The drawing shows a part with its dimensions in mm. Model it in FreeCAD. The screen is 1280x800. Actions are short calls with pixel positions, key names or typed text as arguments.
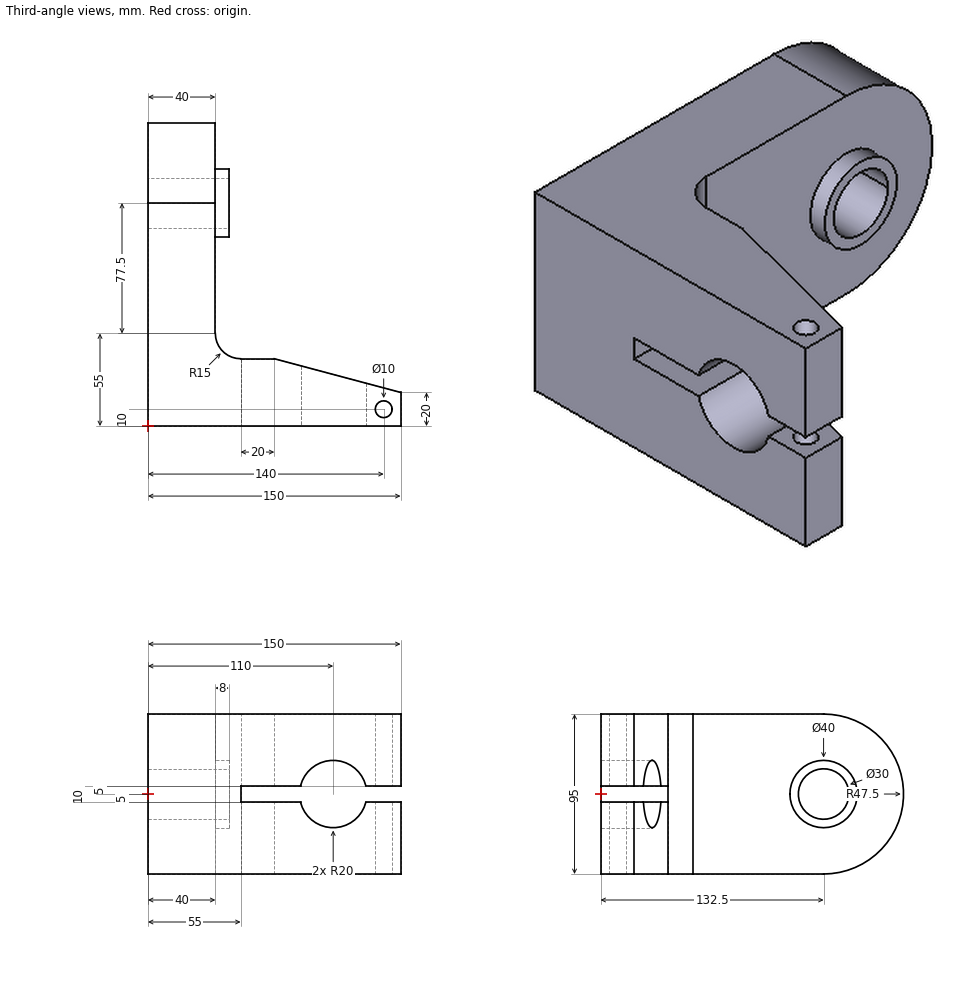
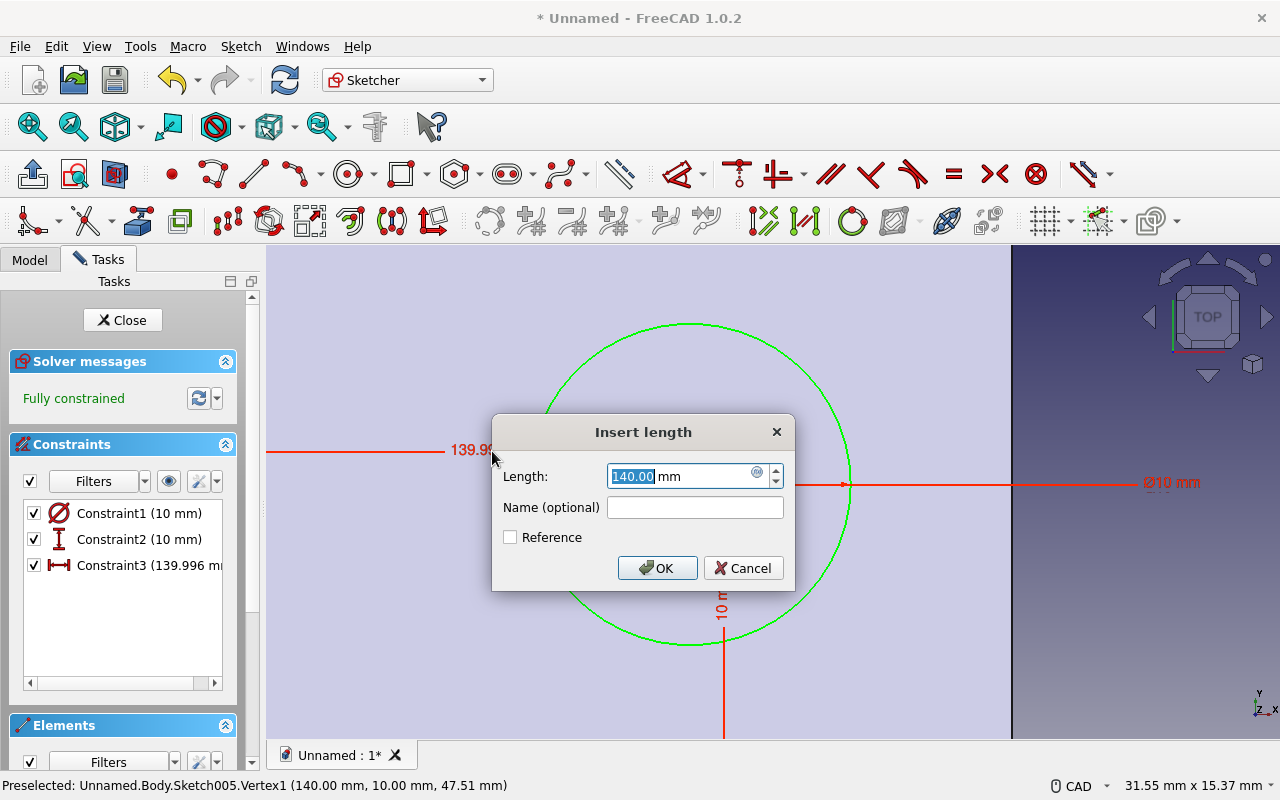
text(140)
key(Return)
key(Escape)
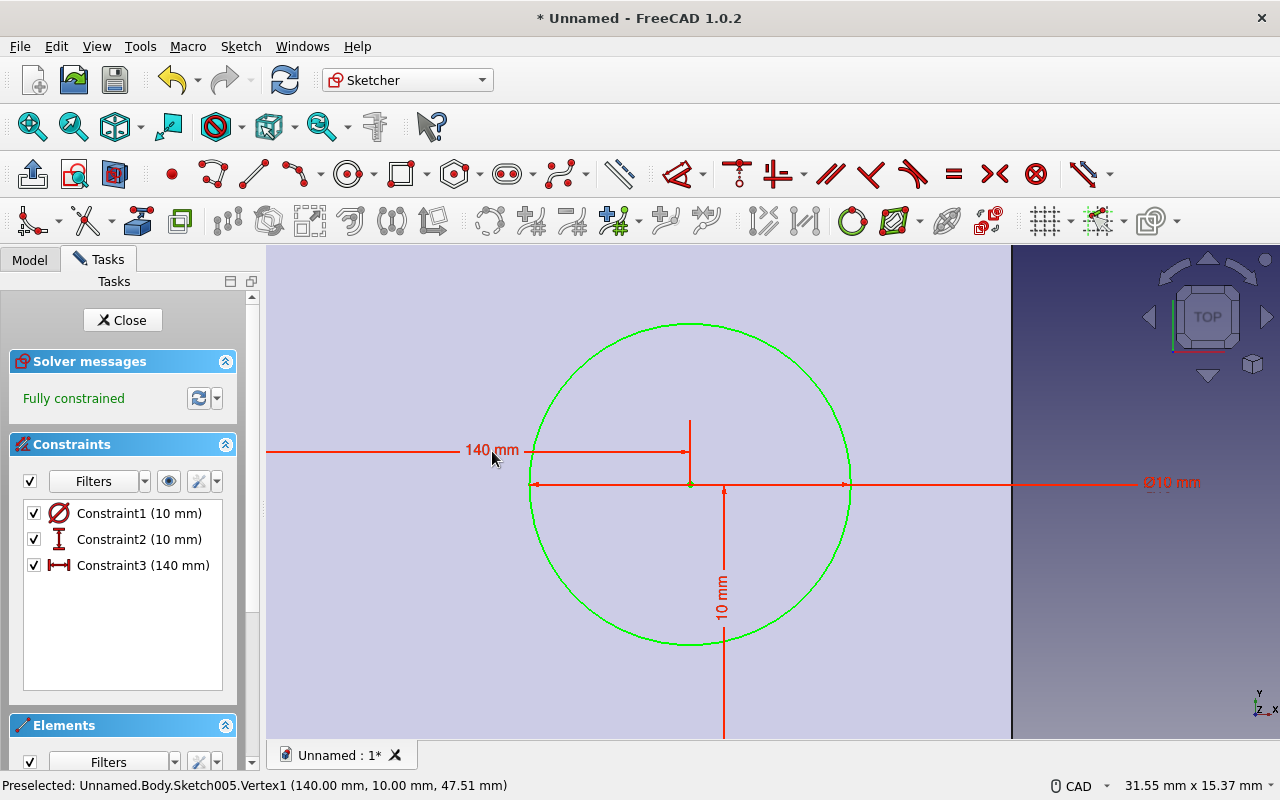
click(123, 320)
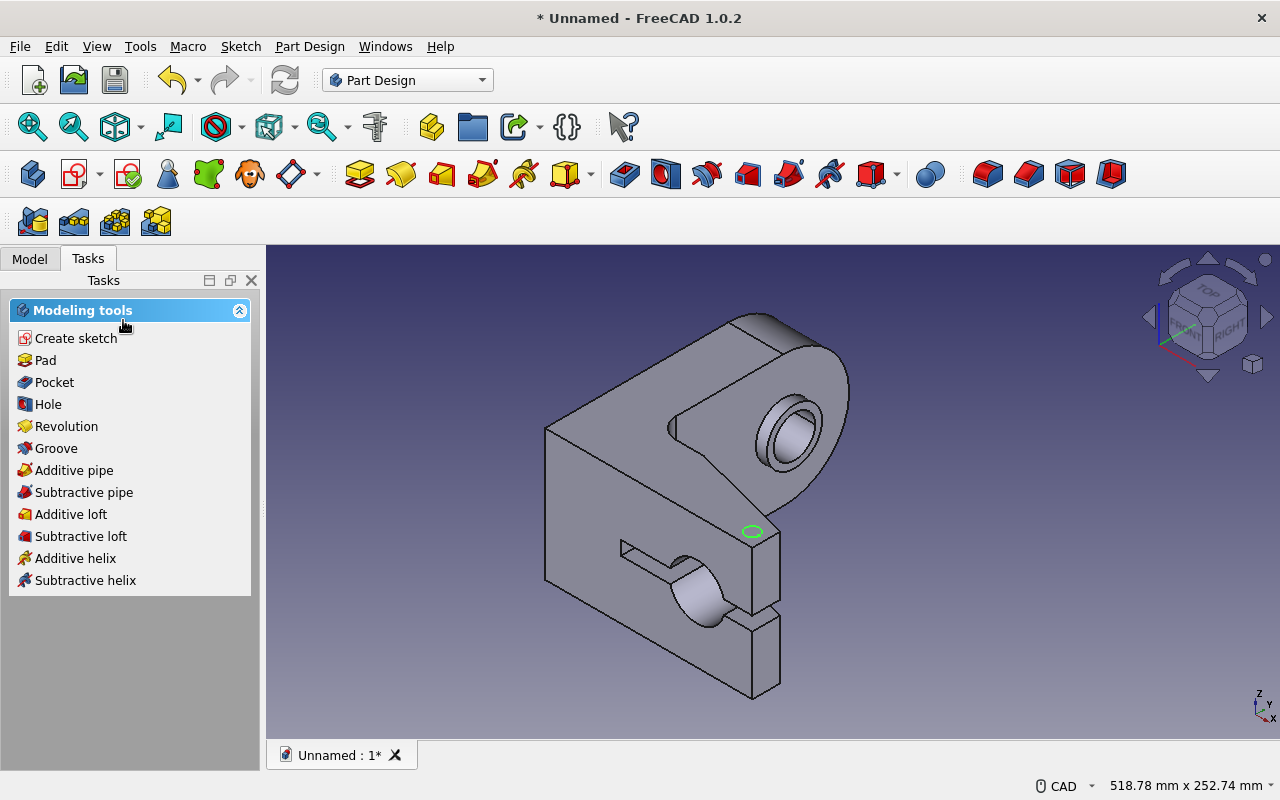
click(625, 174)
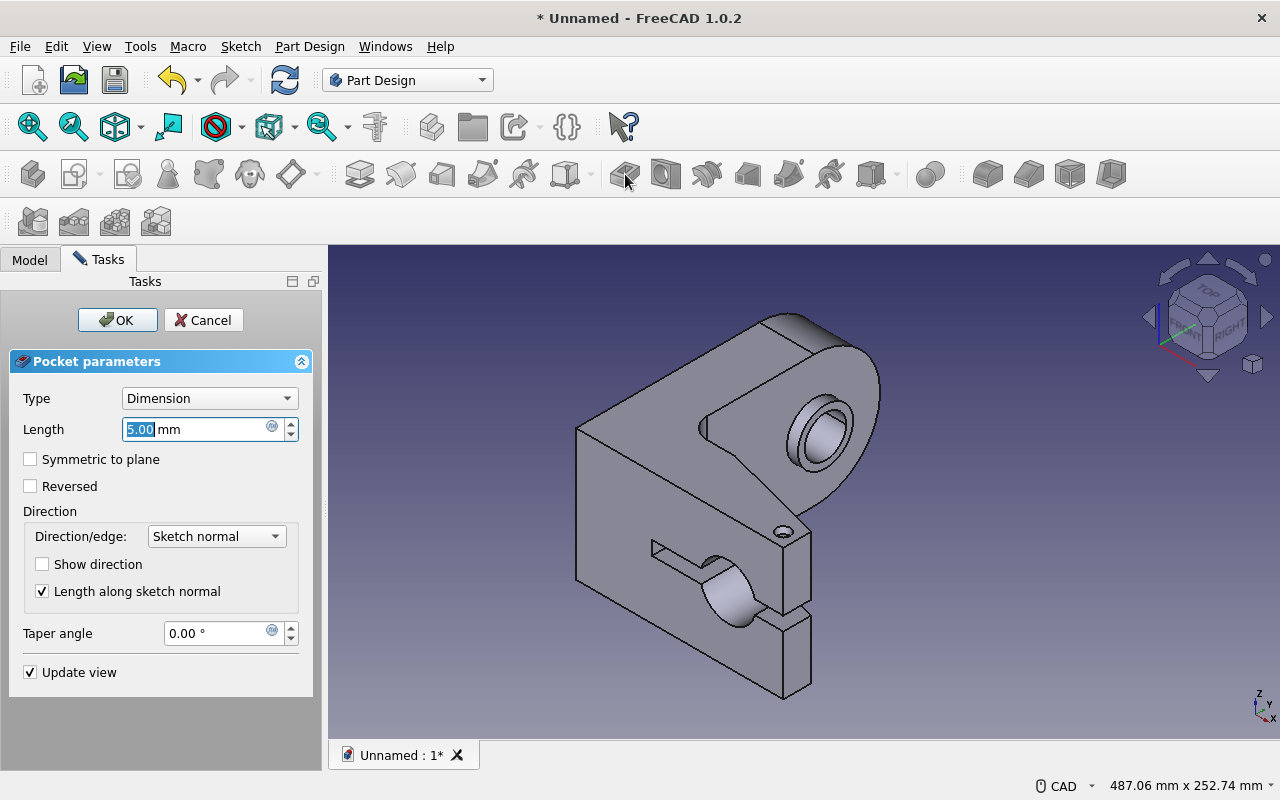
click(210, 398)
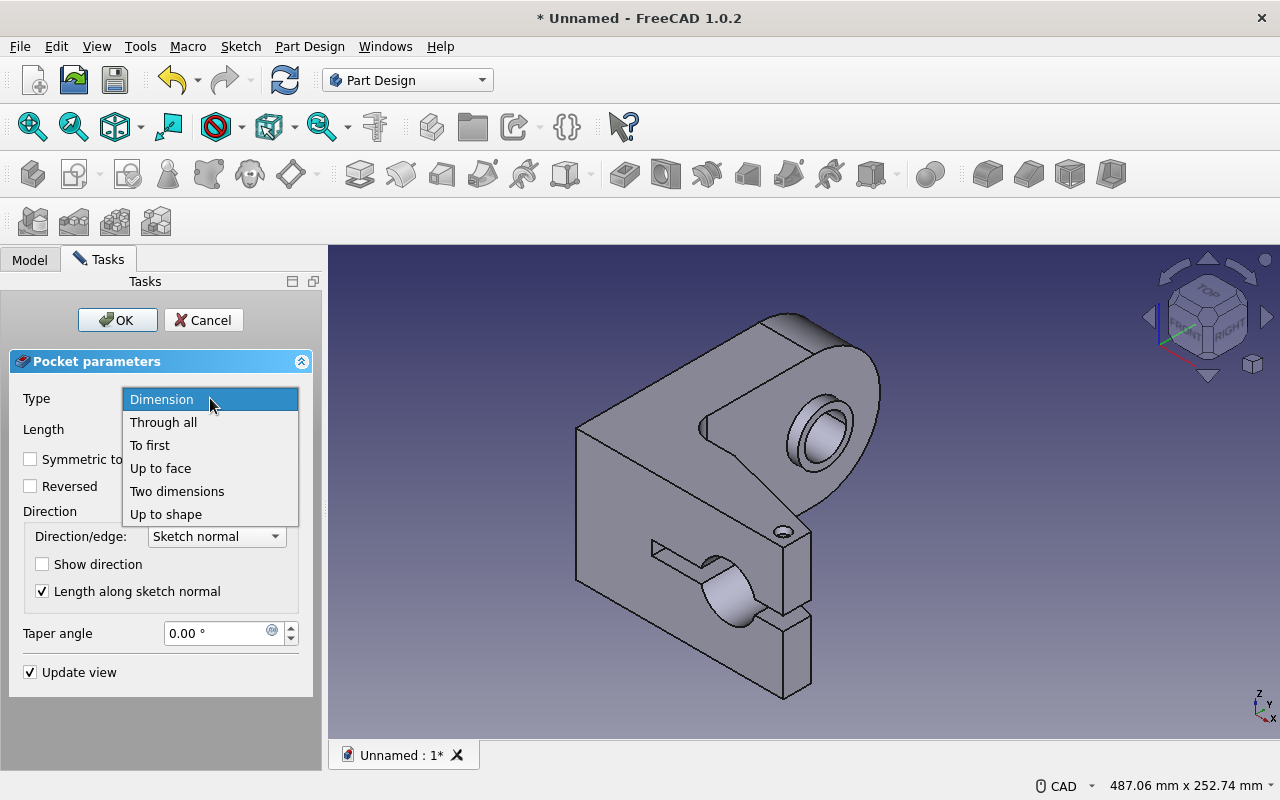
click(208, 422)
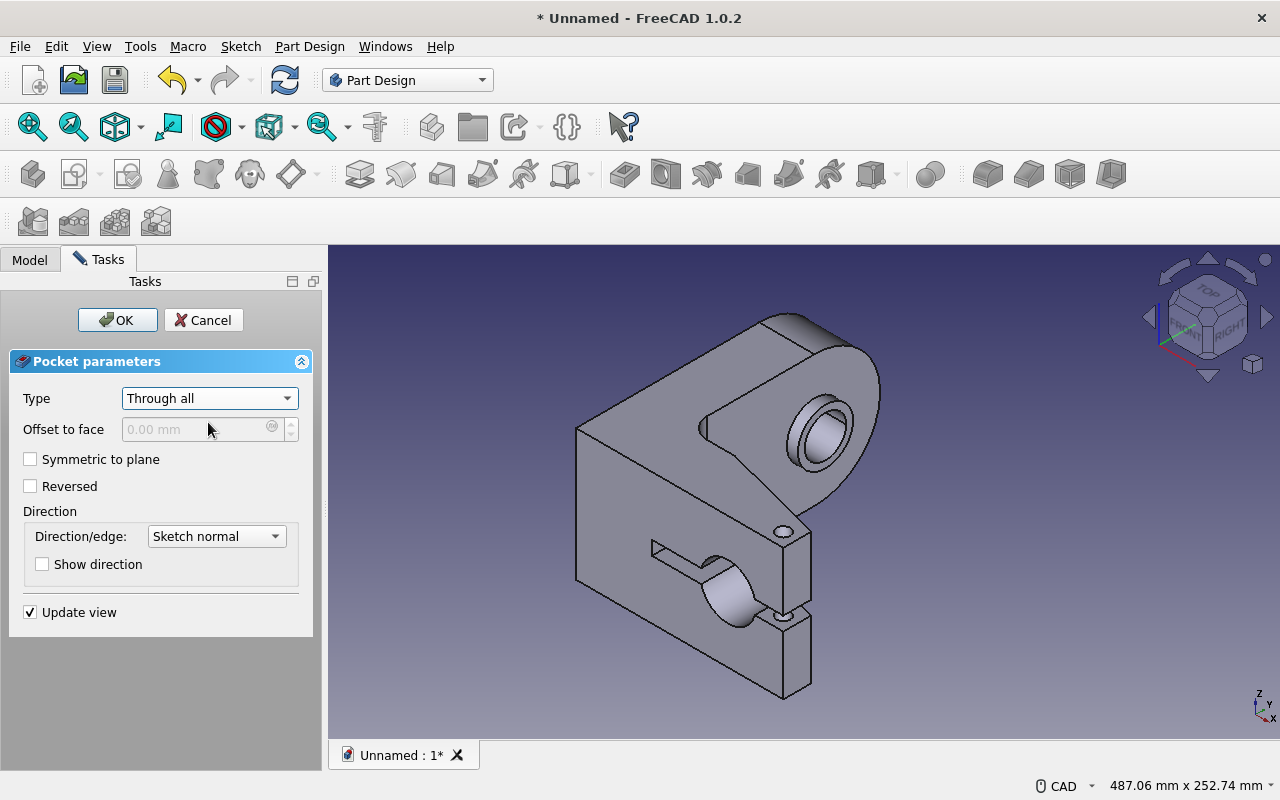
click(118, 320)